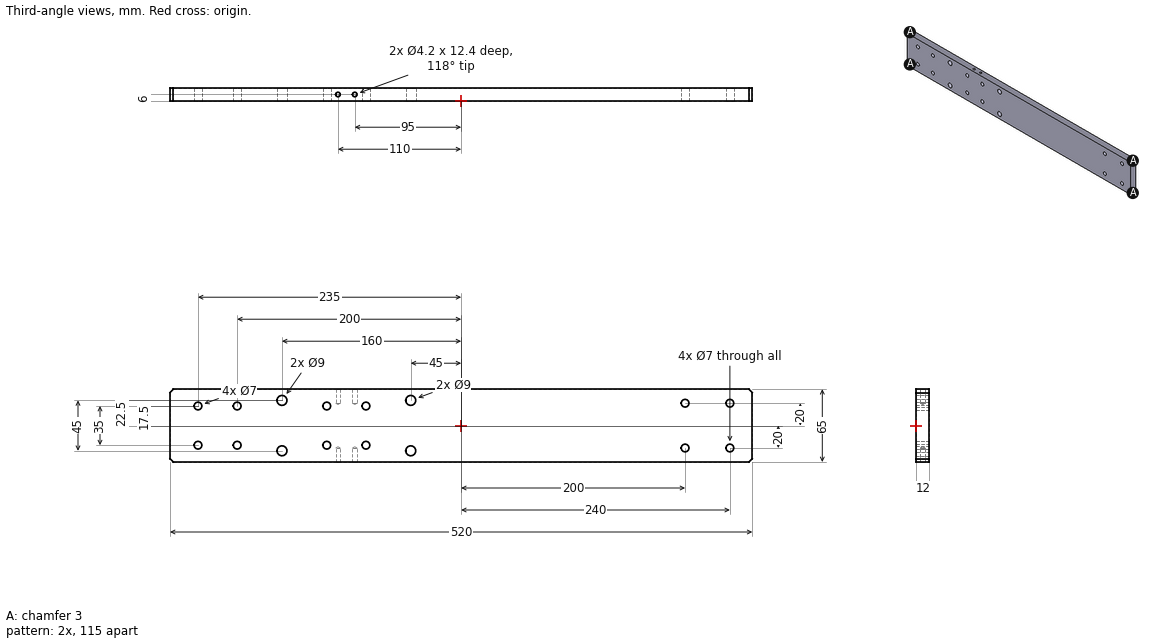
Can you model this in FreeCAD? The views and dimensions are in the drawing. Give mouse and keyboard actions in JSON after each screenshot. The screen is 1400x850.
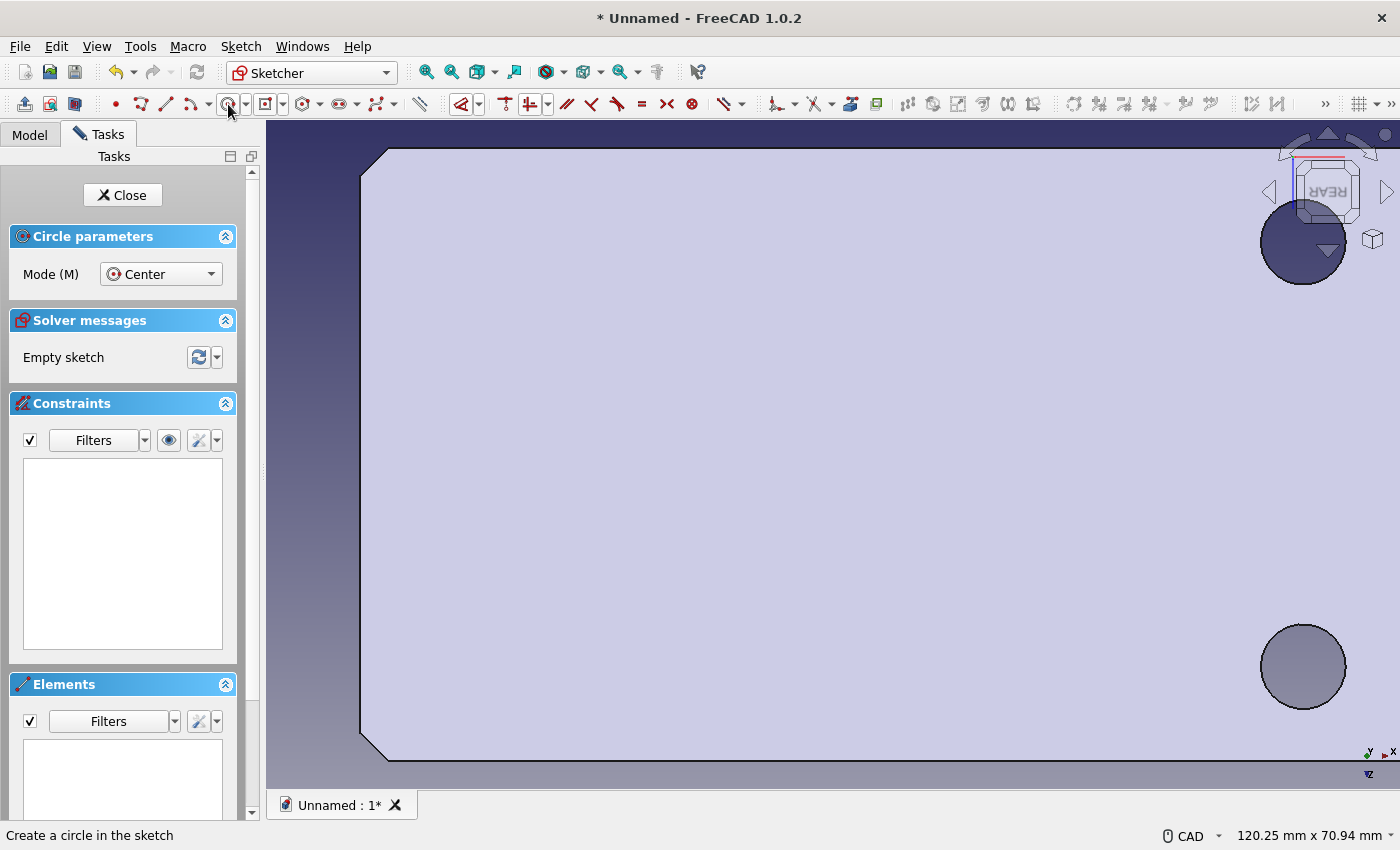
{"action": "left_click", "coordinate": [596, 620]}
{"action": "left_click", "coordinate": [619, 596]}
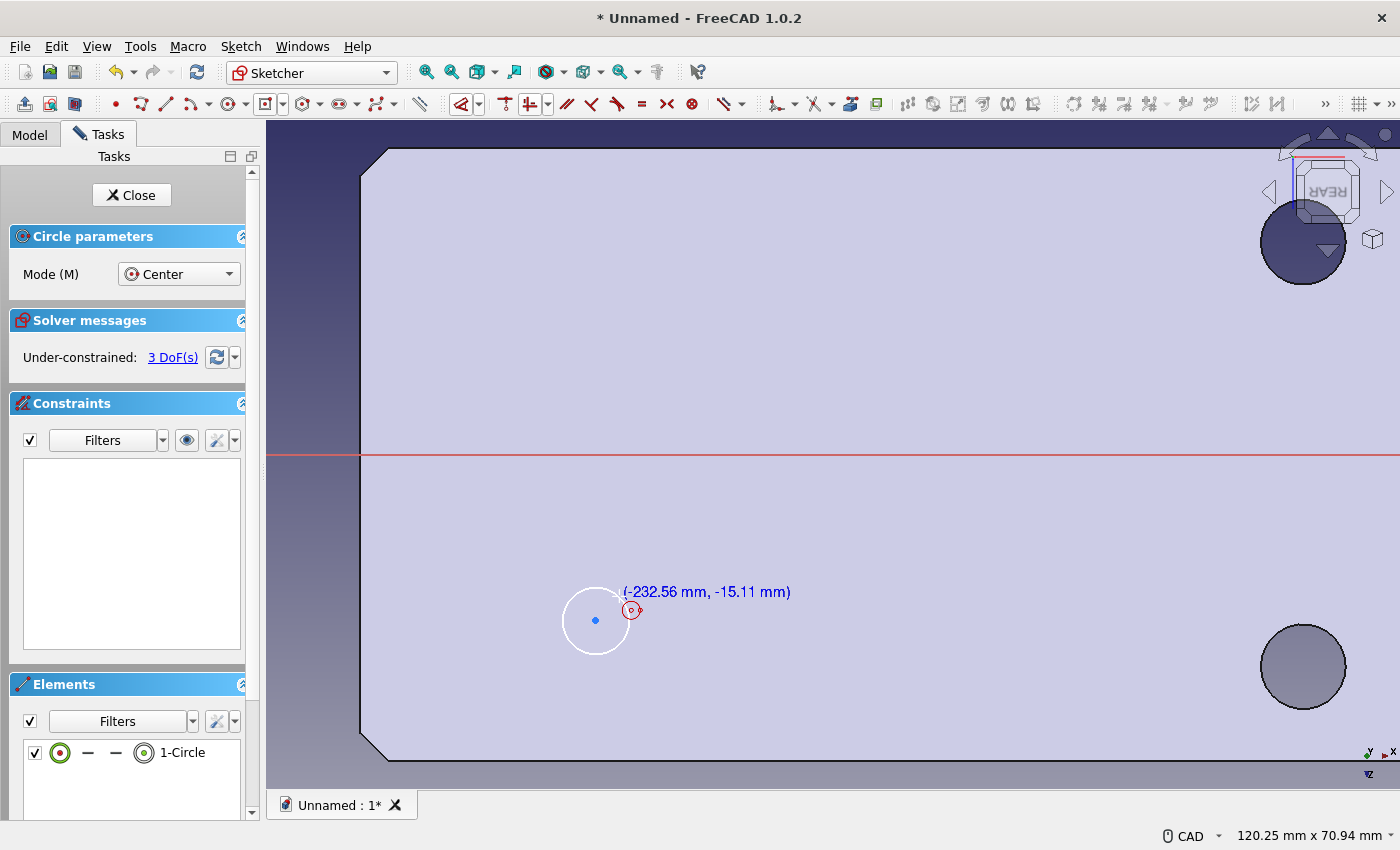
{"action": "left_click", "coordinate": [596, 289]}
{"action": "left_click", "coordinate": [619, 266]}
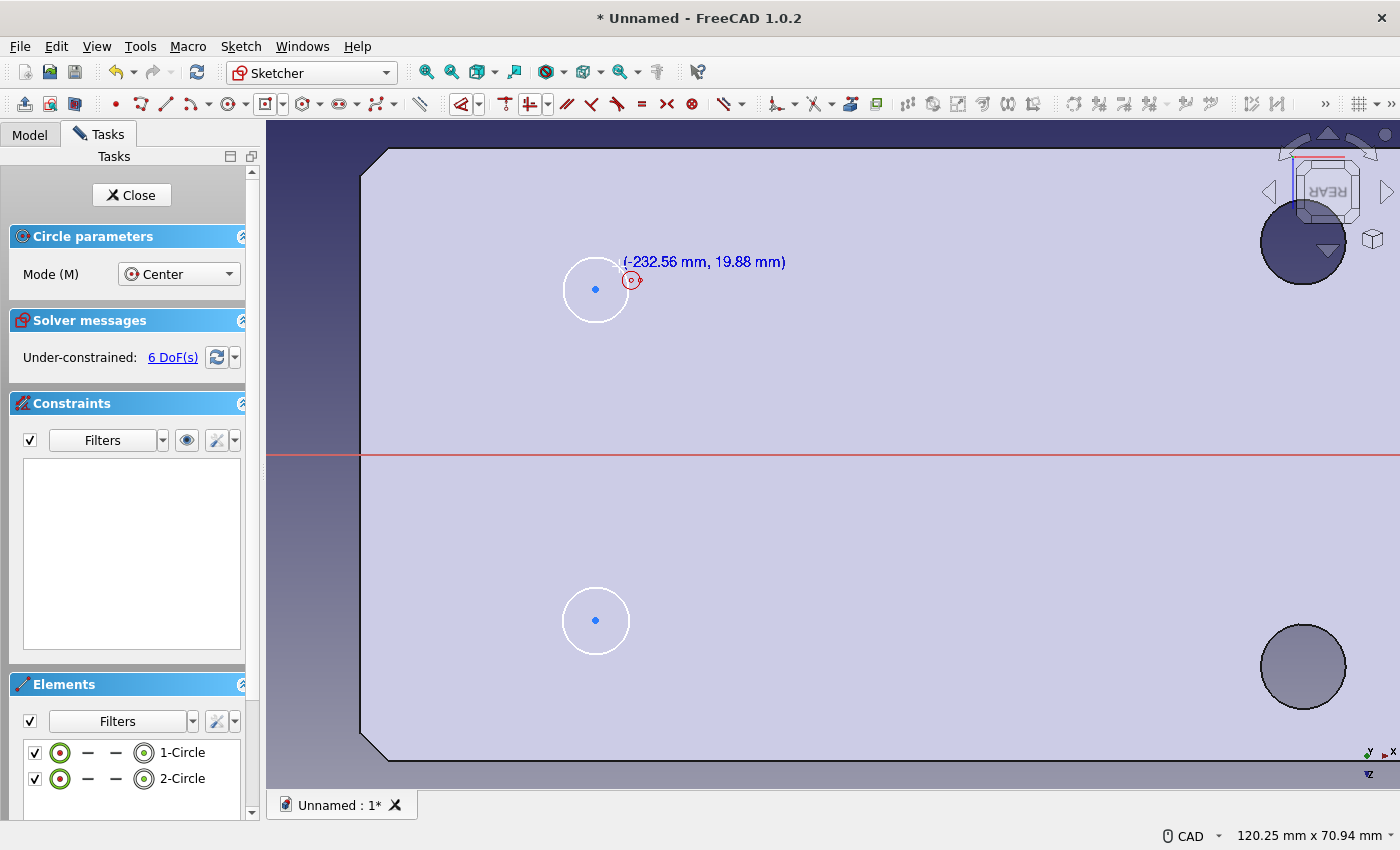
{"action": "left_click", "coordinate": [926, 620]}
{"action": "left_click", "coordinate": [949, 596]}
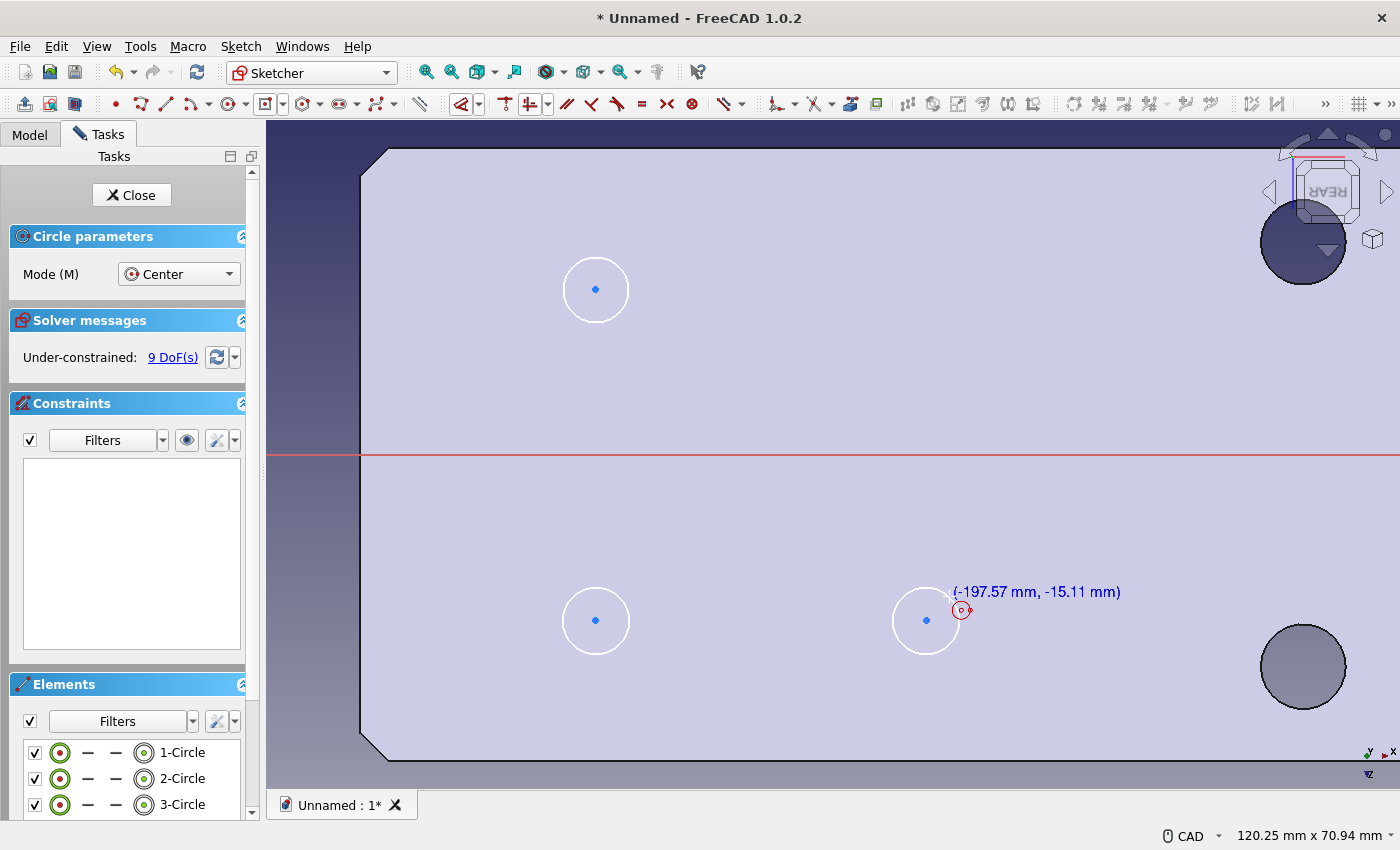
{"action": "left_click", "coordinate": [926, 289]}
{"action": "left_click", "coordinate": [949, 266]}
{"action": "key", "text": "Escape"}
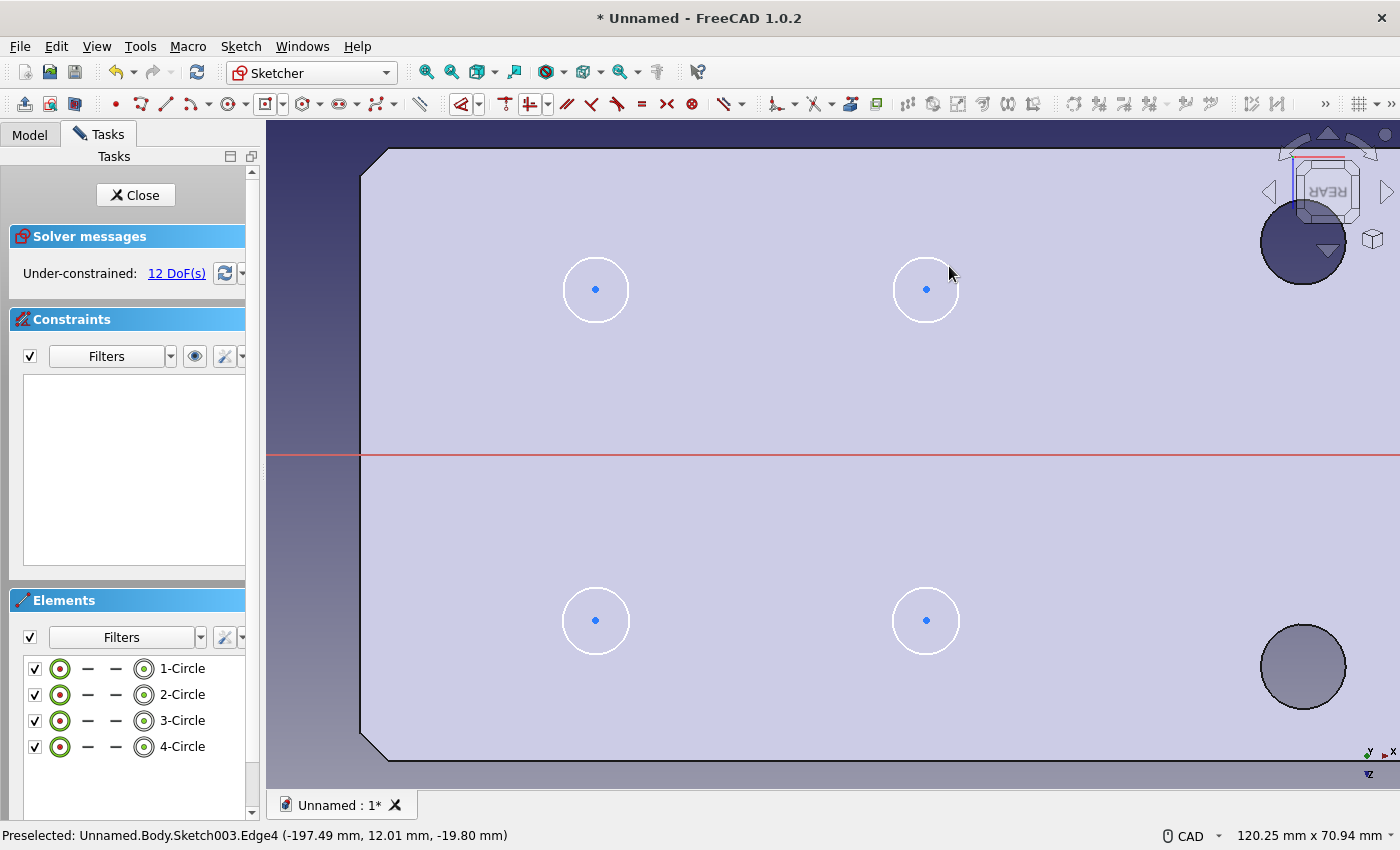
{"action": "left_click", "coordinate": [619, 597]}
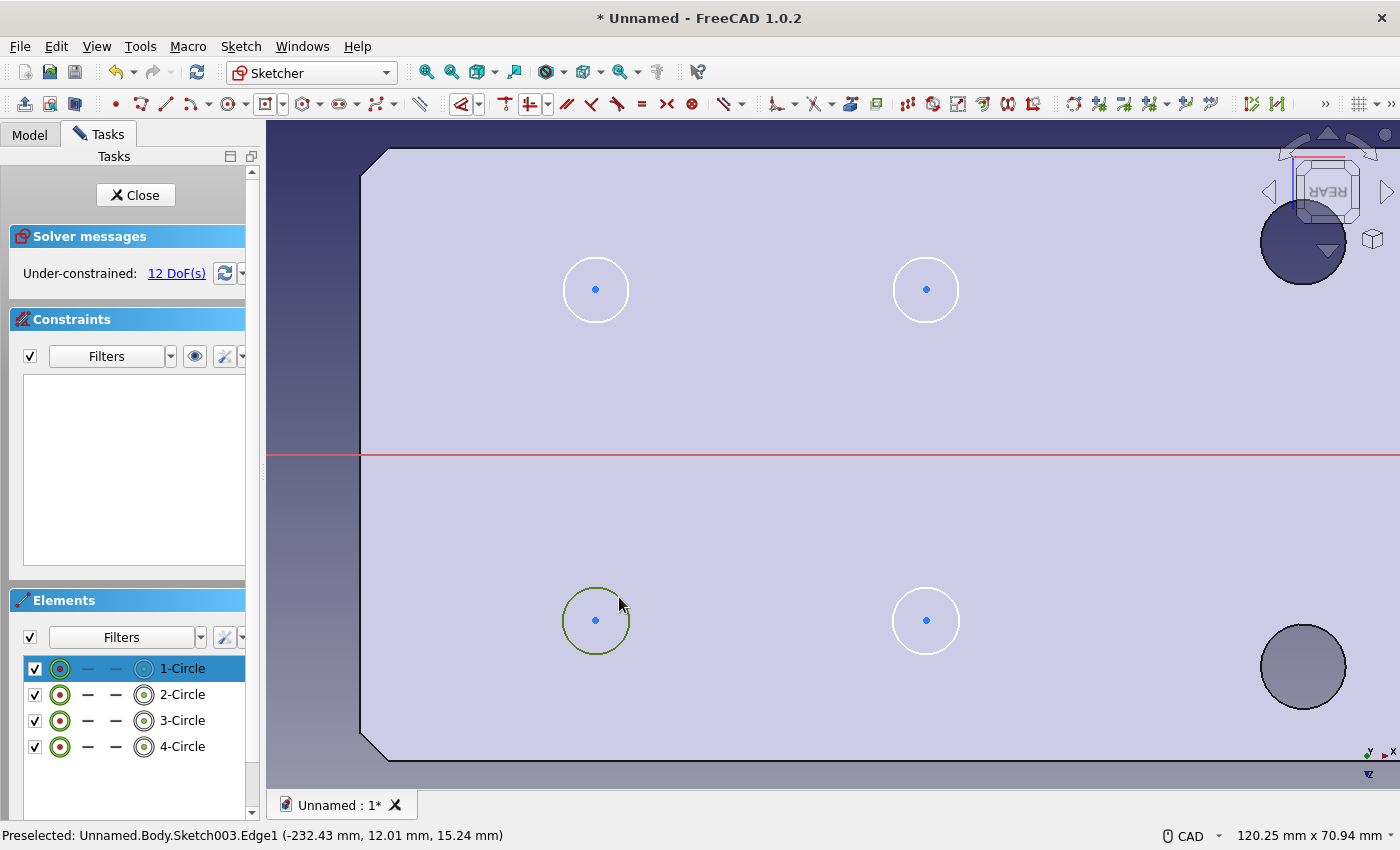
{"action": "left_click", "coordinate": [619, 267]}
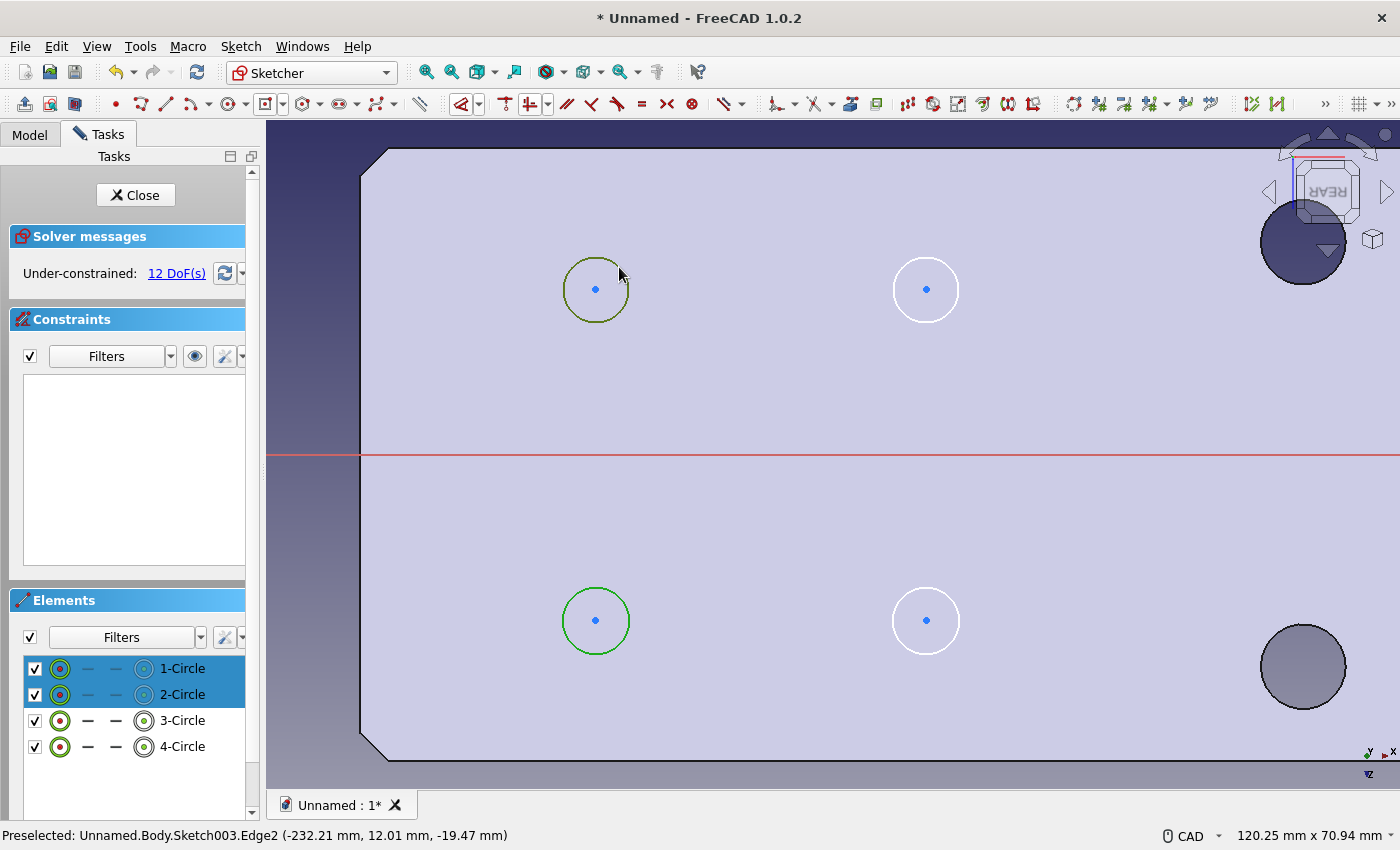
{"action": "left_click", "coordinate": [949, 597]}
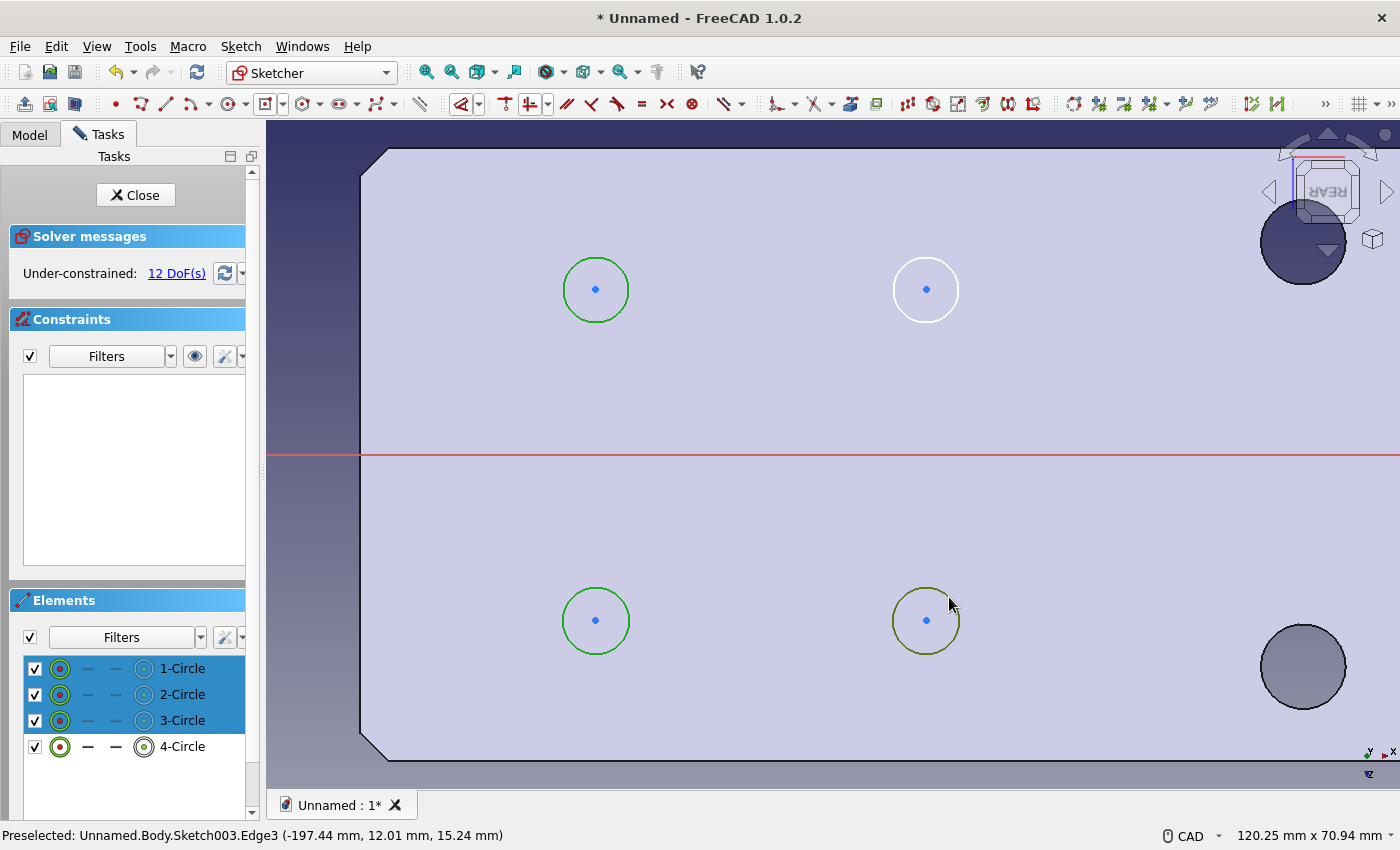
{"action": "left_click", "coordinate": [949, 267]}